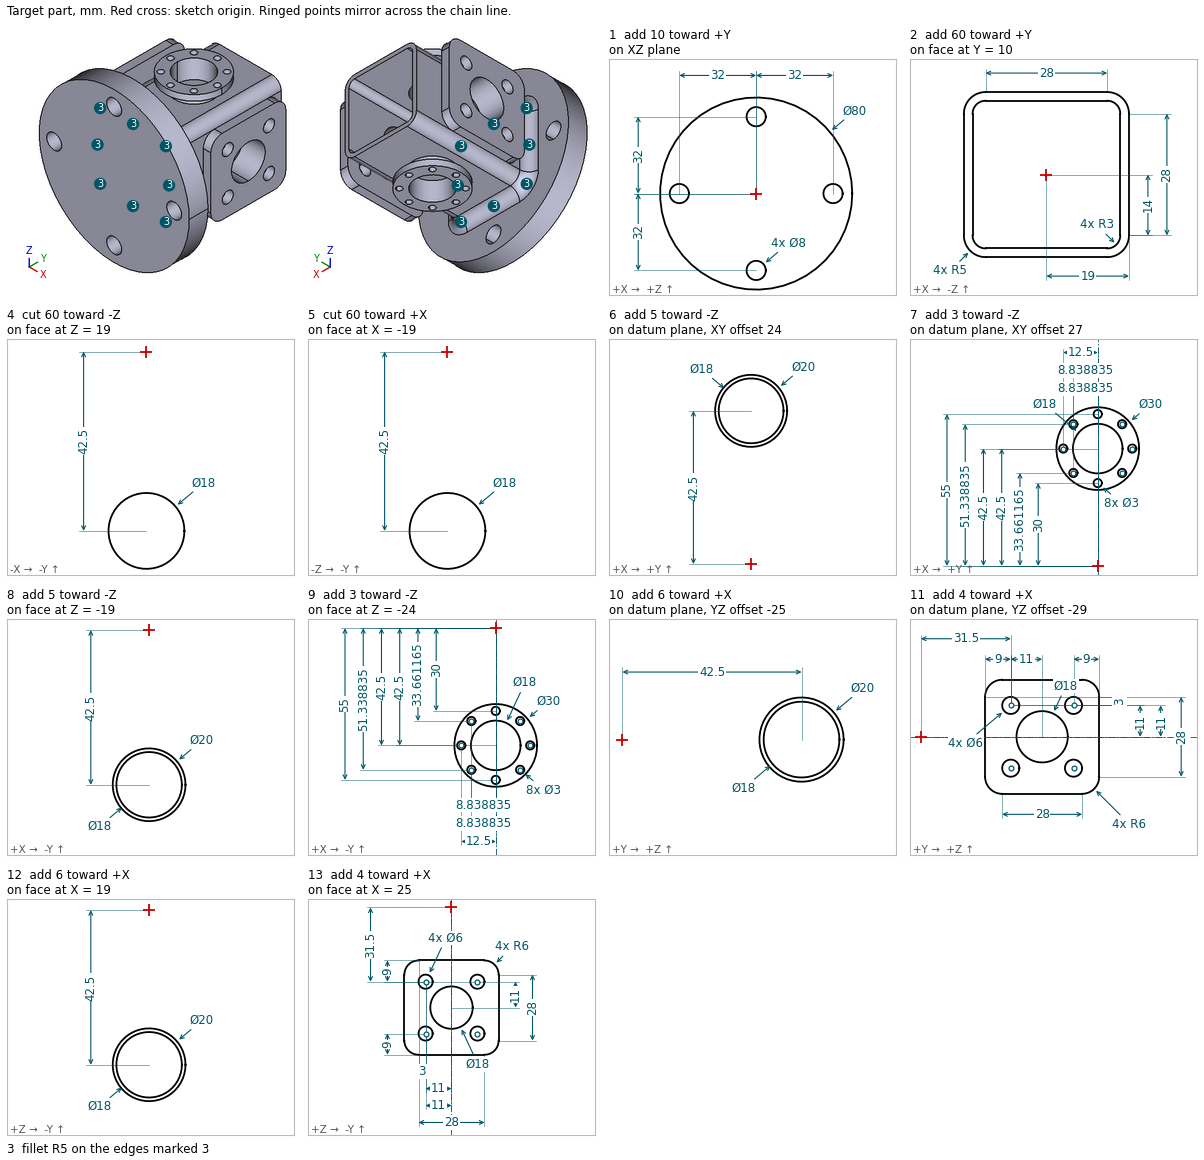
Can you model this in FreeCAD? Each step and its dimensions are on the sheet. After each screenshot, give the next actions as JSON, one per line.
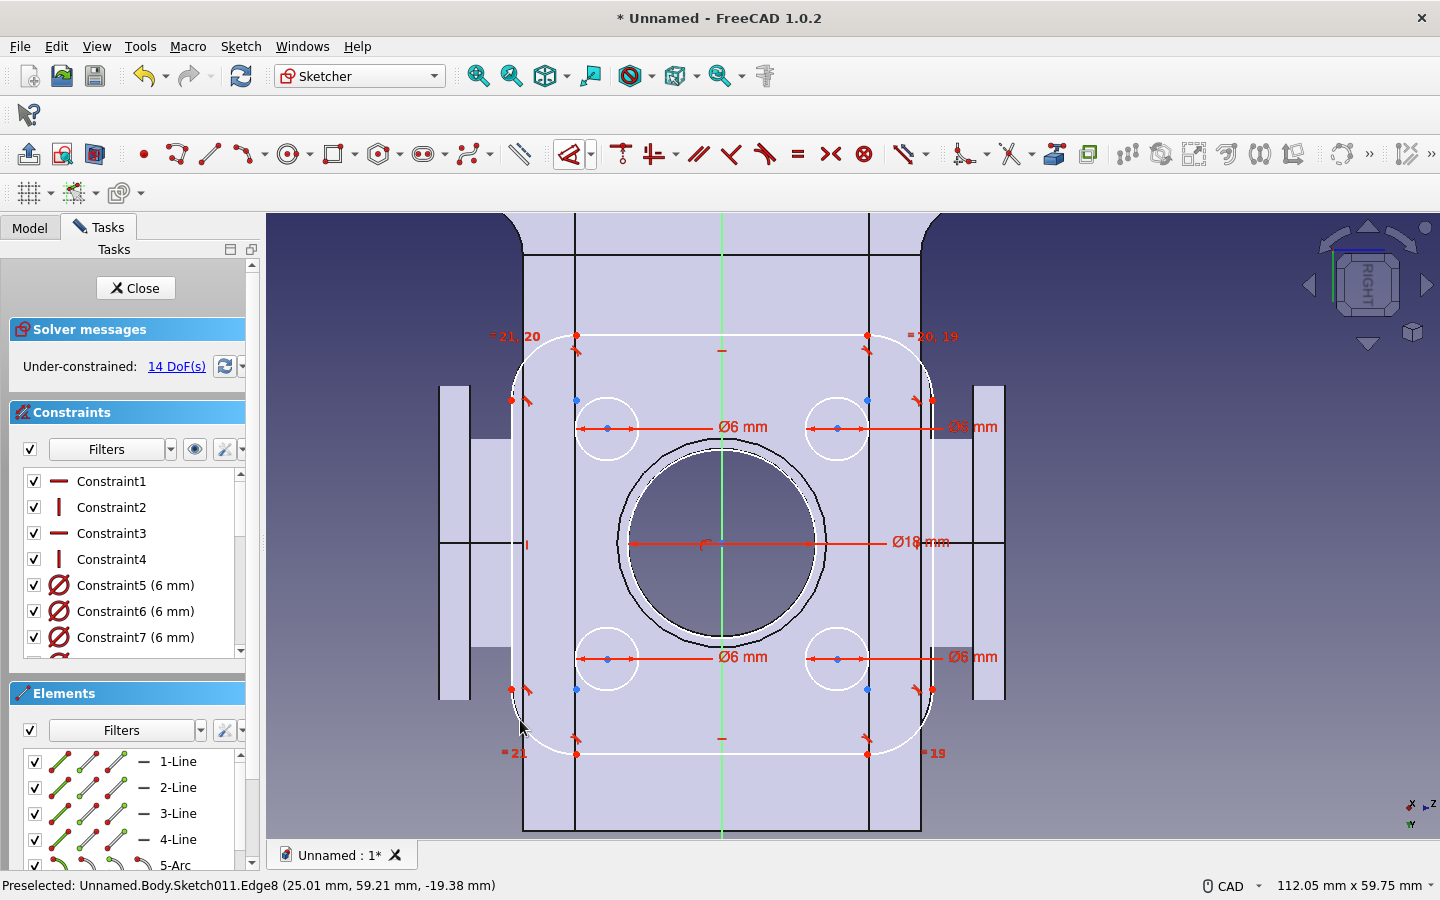
{"action": "left_click", "coordinate": [607, 429]}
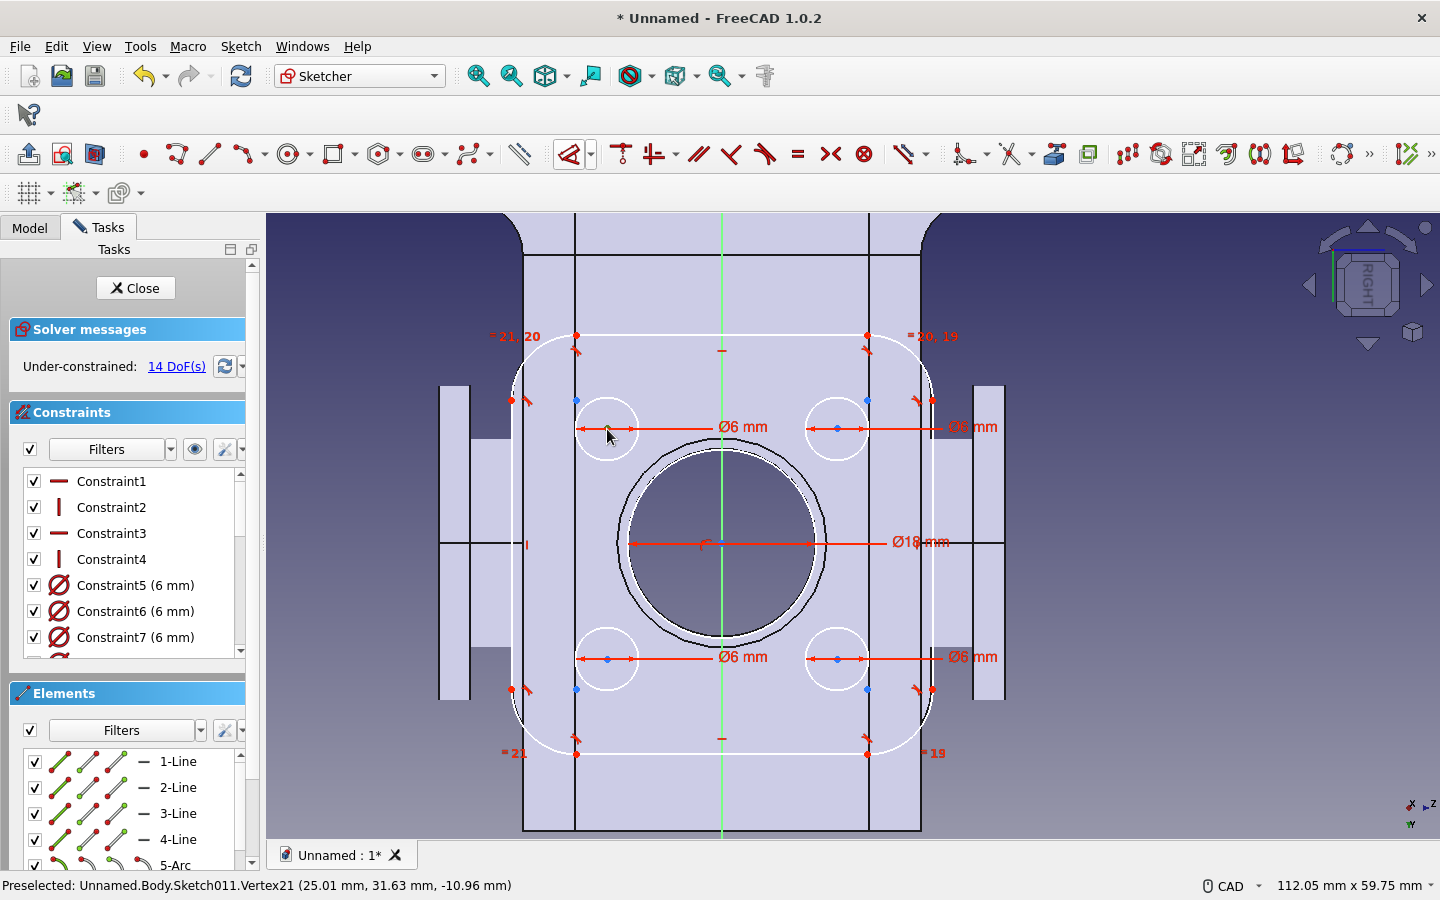
{"action": "left_click", "coordinate": [837, 429]}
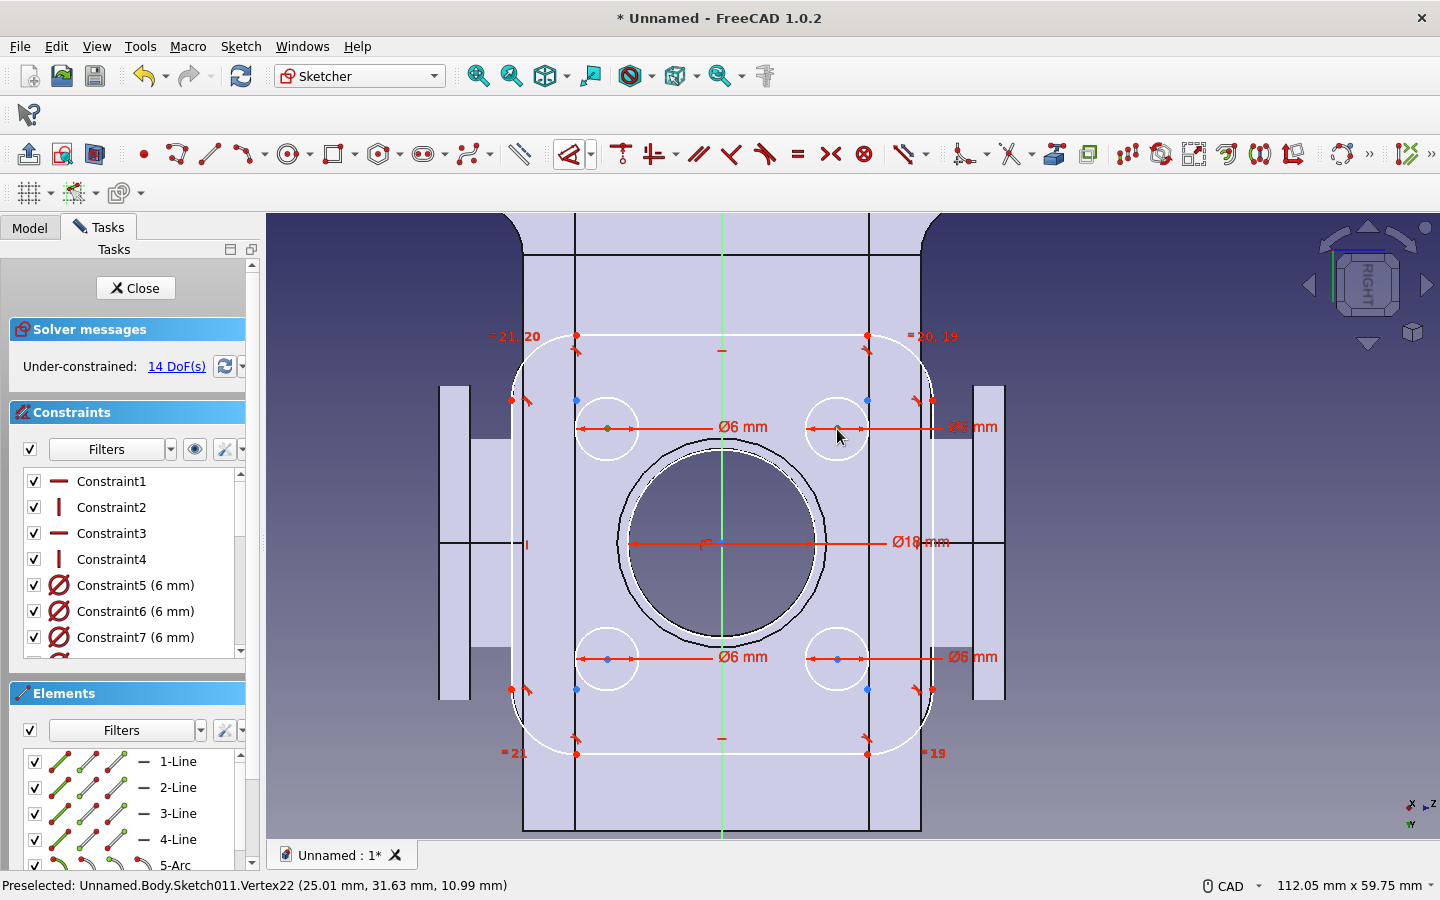
{"action": "left_click", "coordinate": [722, 689]}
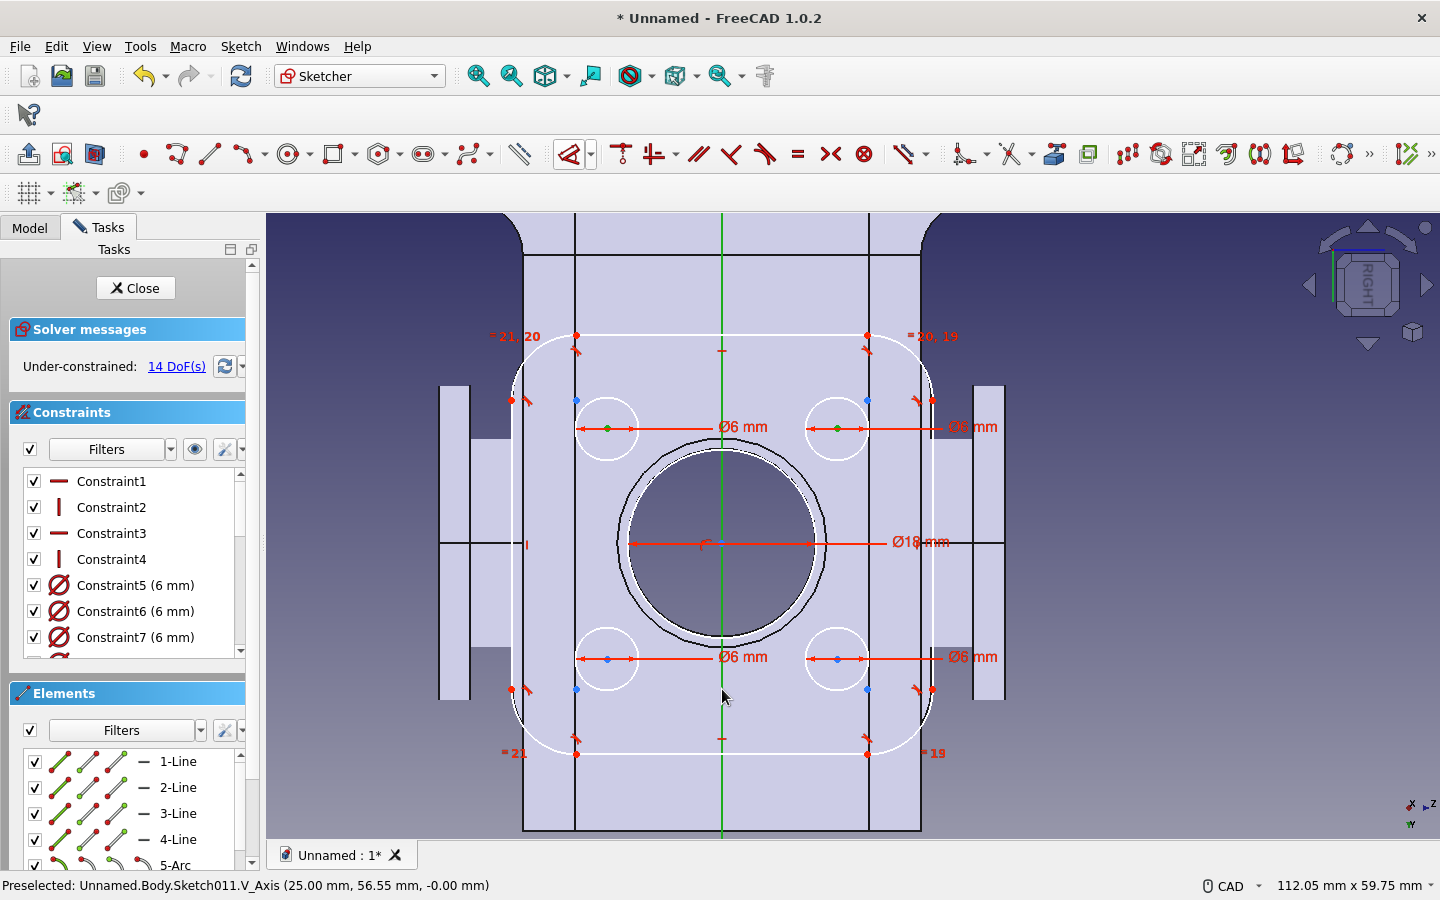
{"action": "key", "text": "s"}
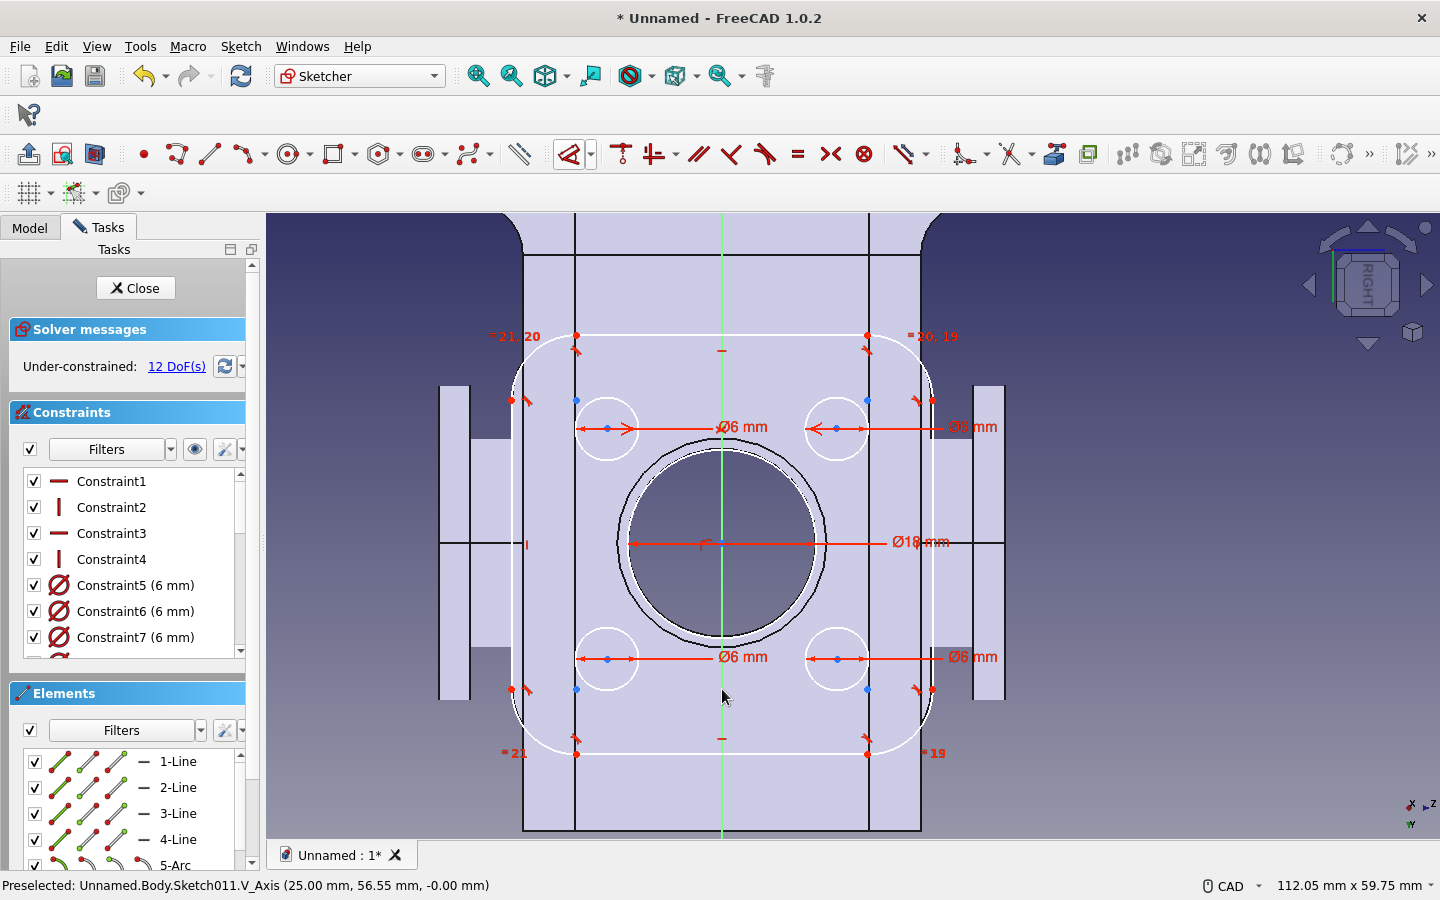
{"action": "left_click", "coordinate": [607, 659]}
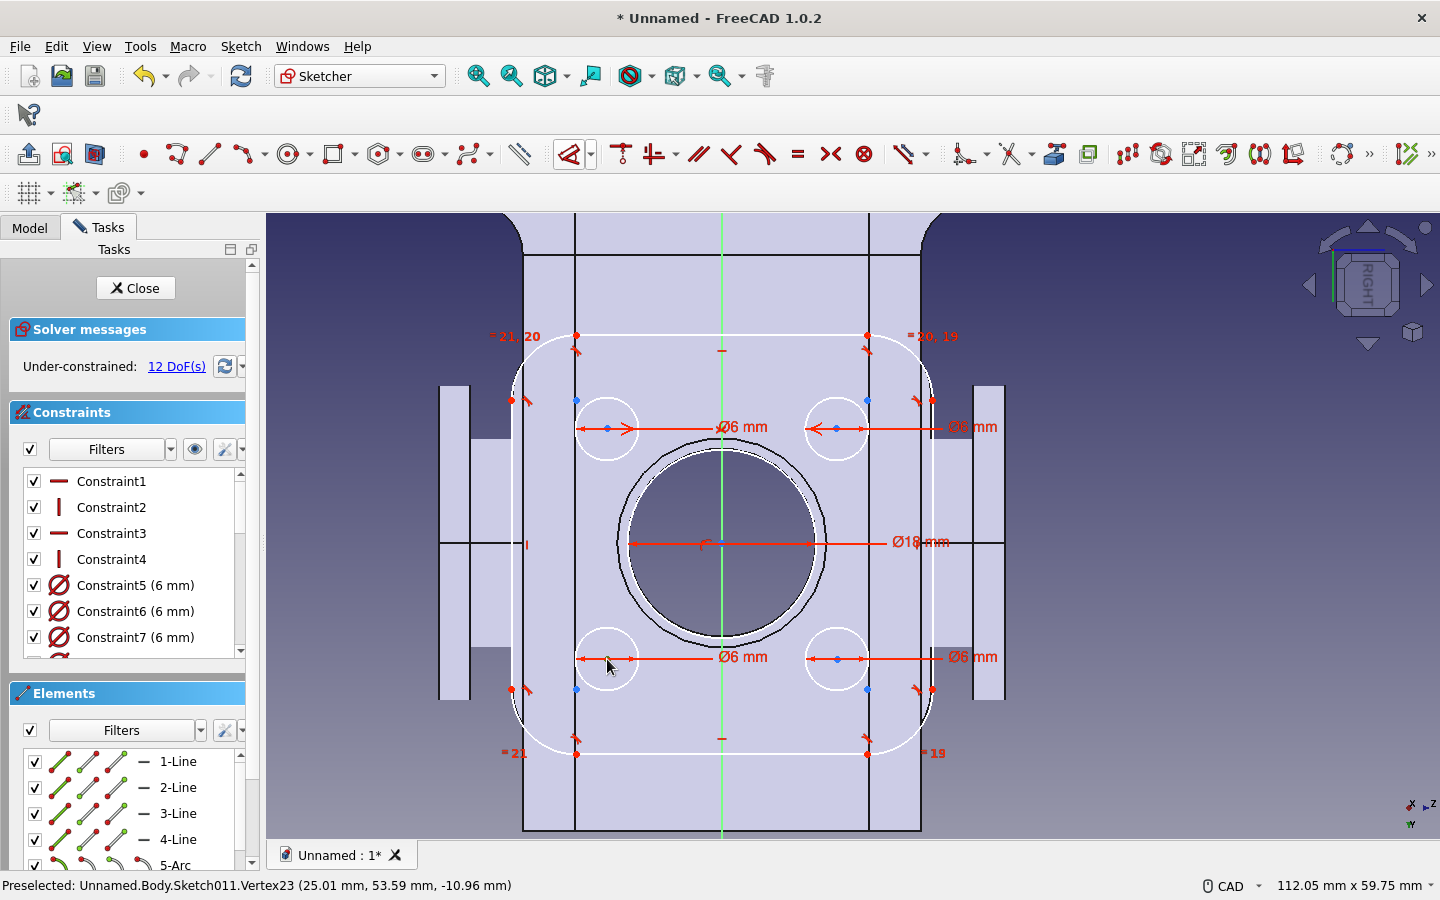
{"action": "left_click", "coordinate": [837, 659]}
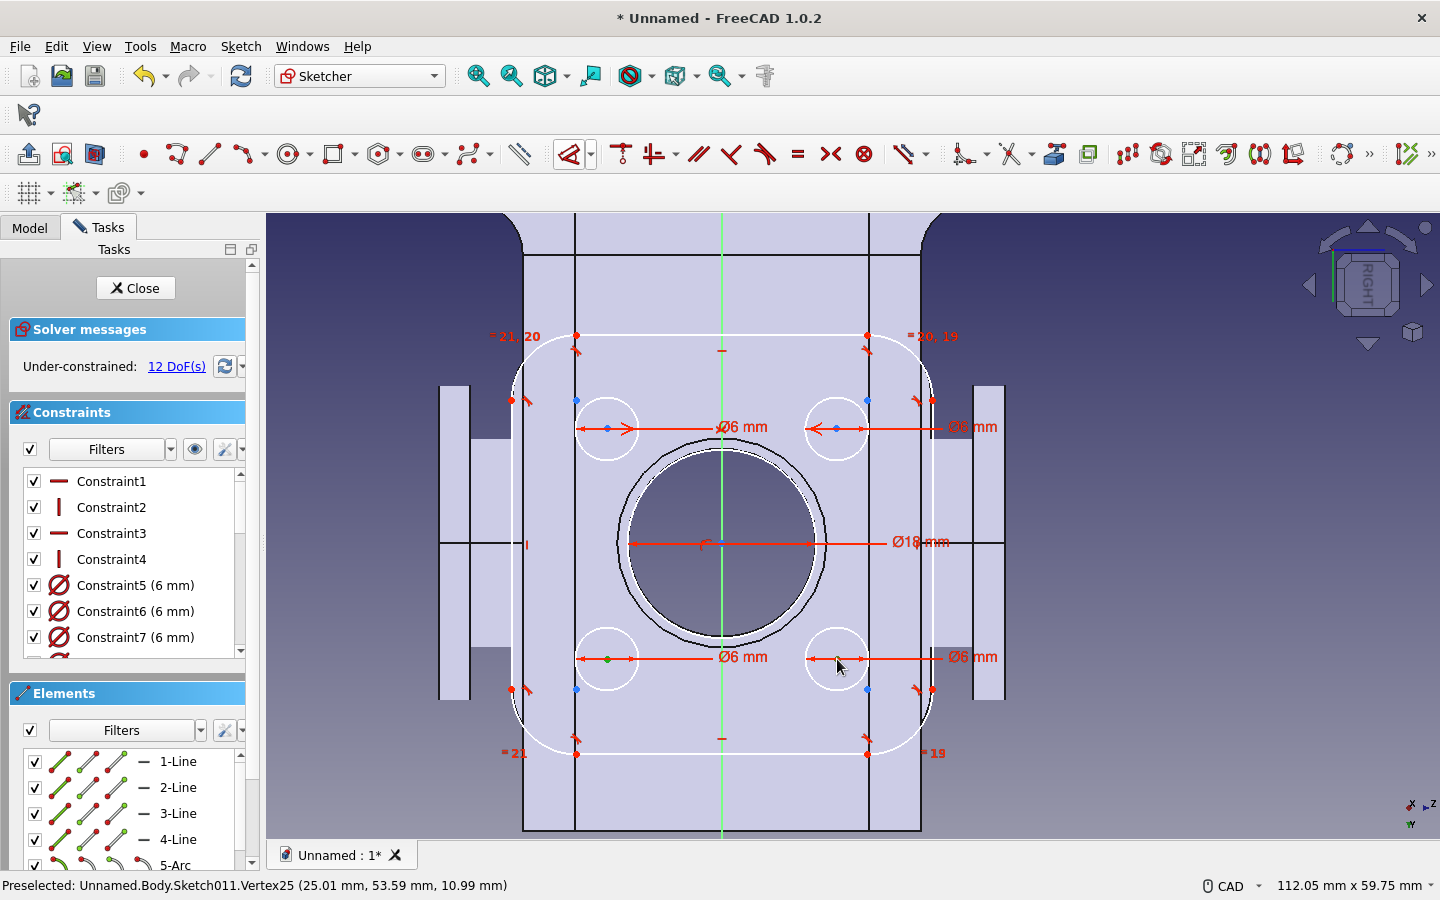
{"action": "left_click", "coordinate": [722, 689]}